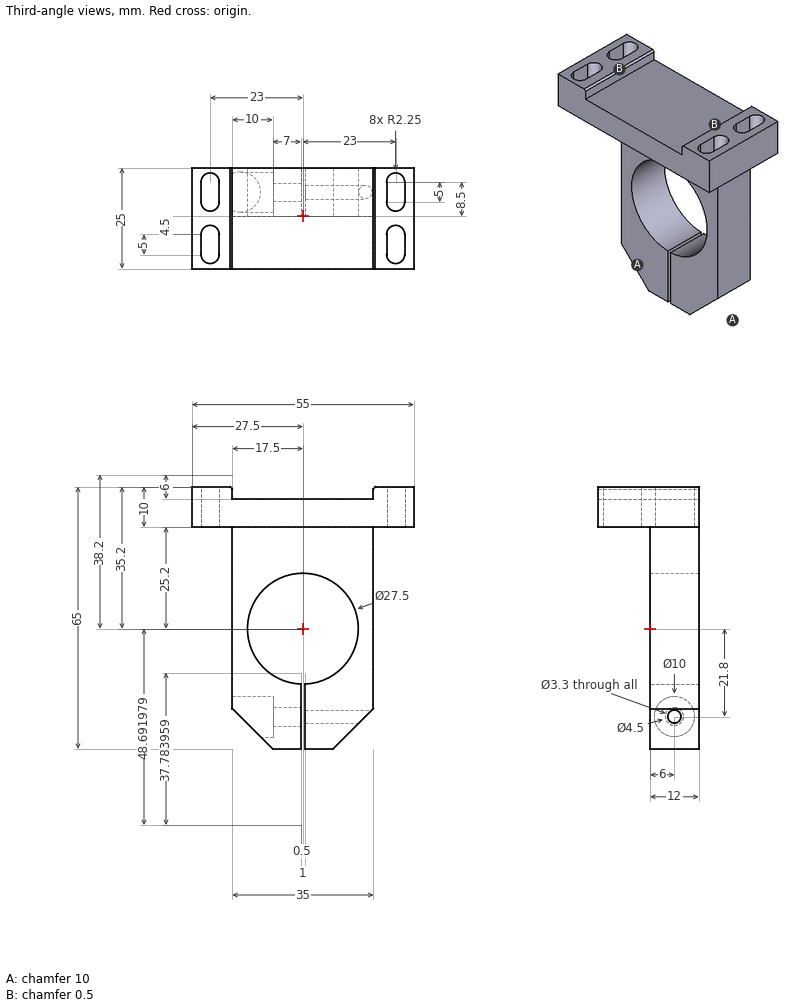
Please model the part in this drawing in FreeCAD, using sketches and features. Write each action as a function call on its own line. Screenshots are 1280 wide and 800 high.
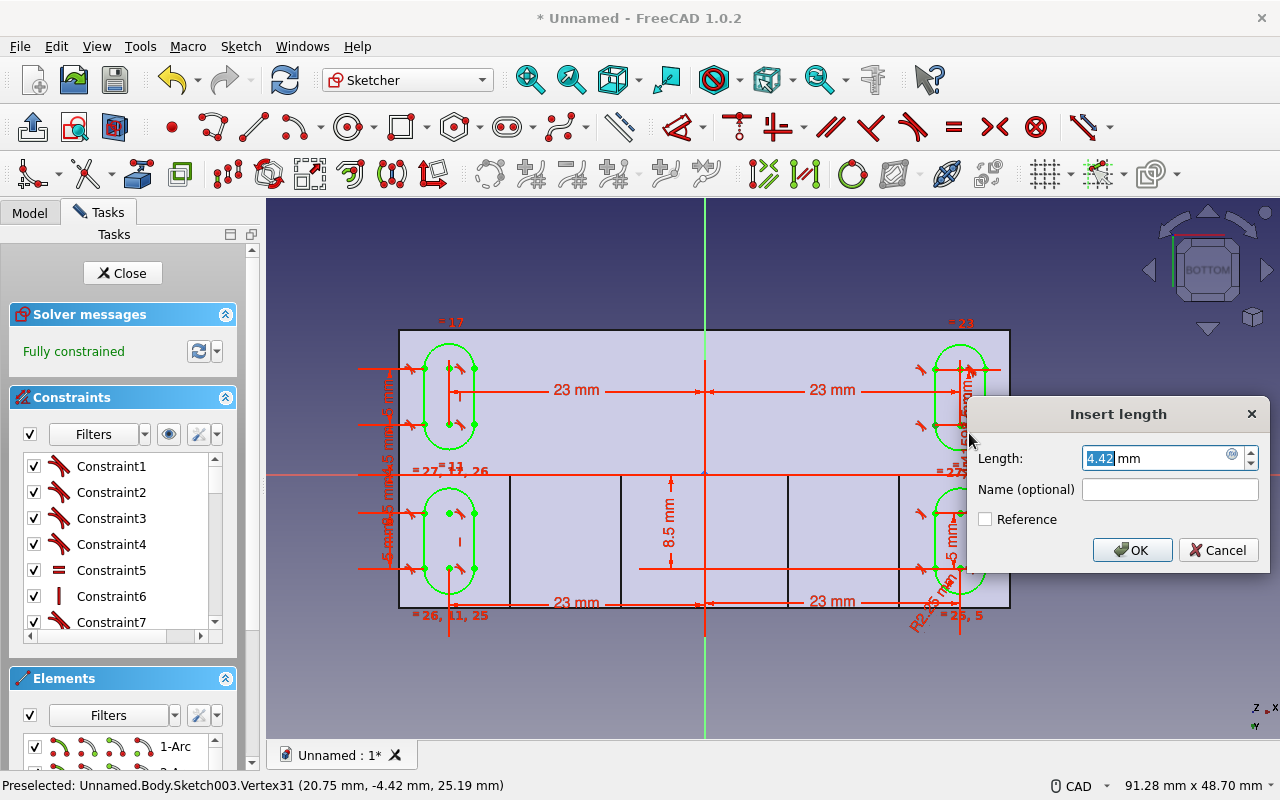
text(4.5)
key(Return)
key(Escape)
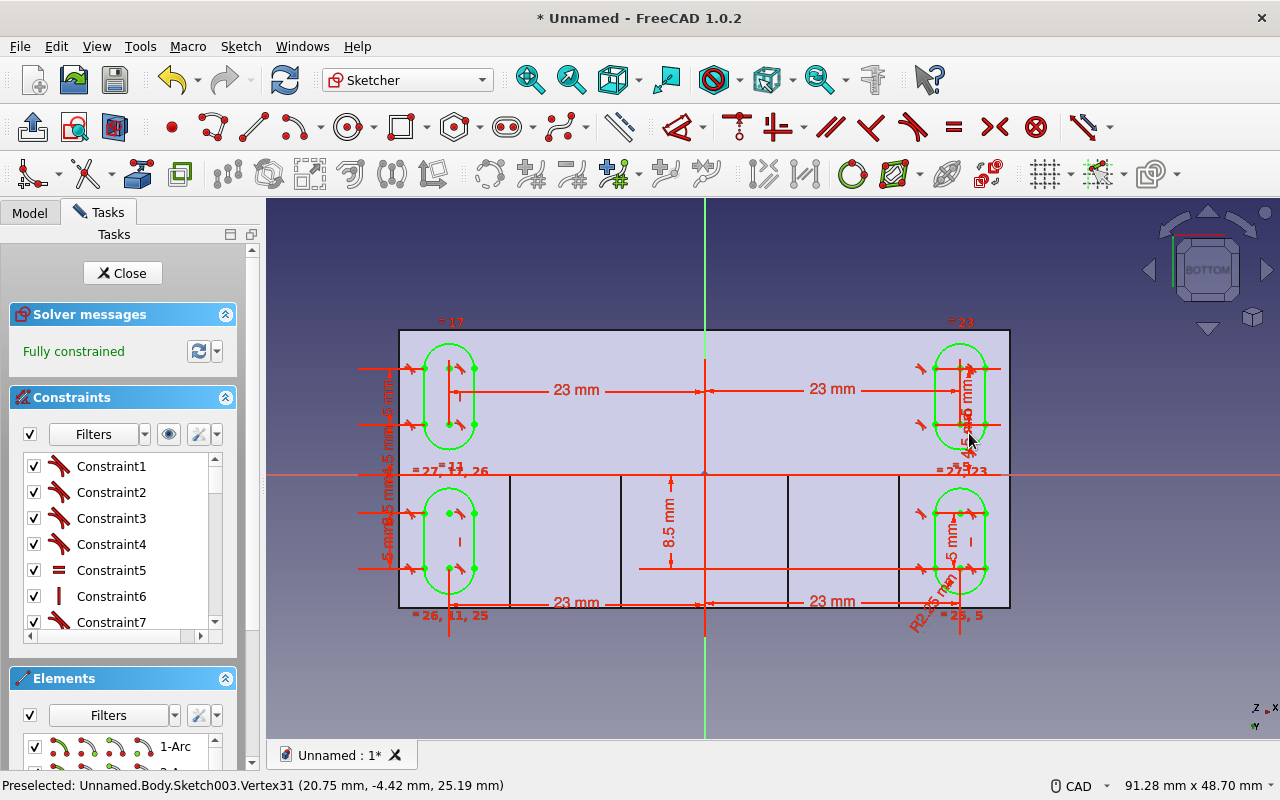
click(123, 273)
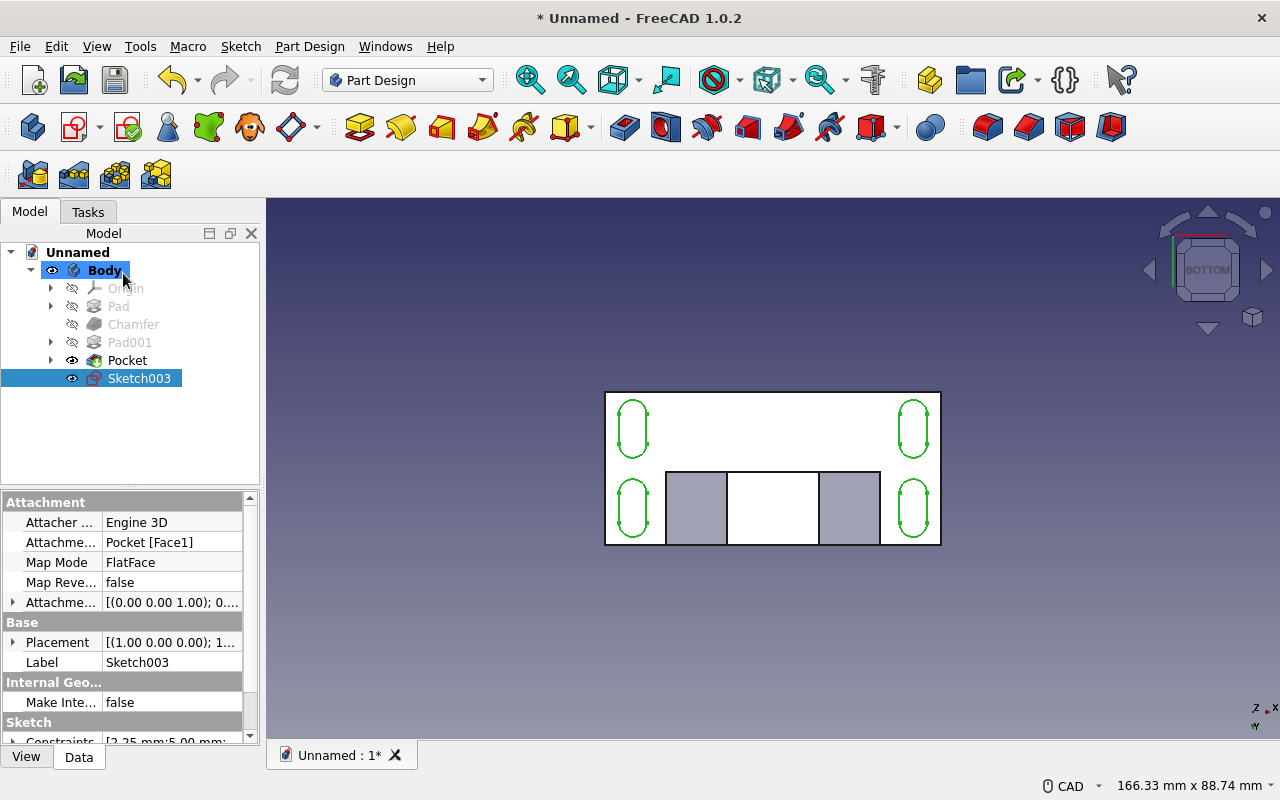
click(625, 128)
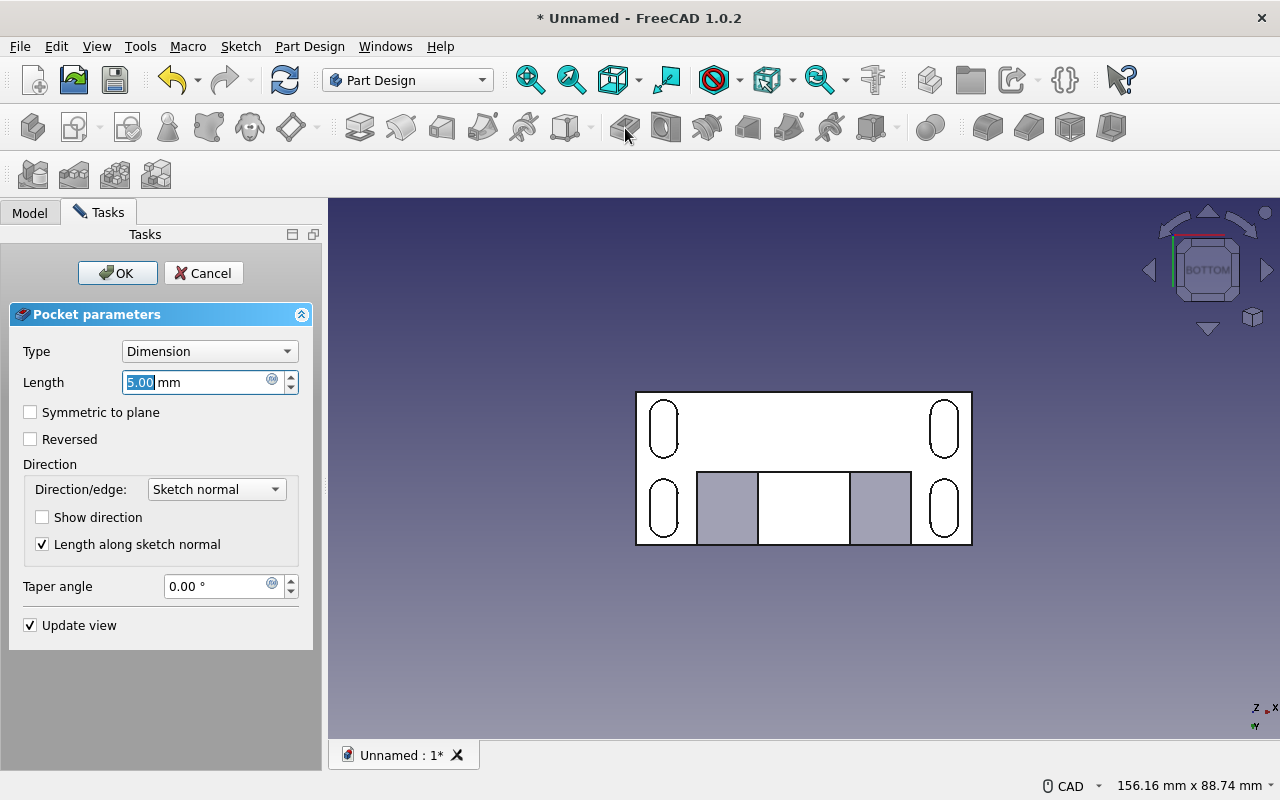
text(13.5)
key(Tab)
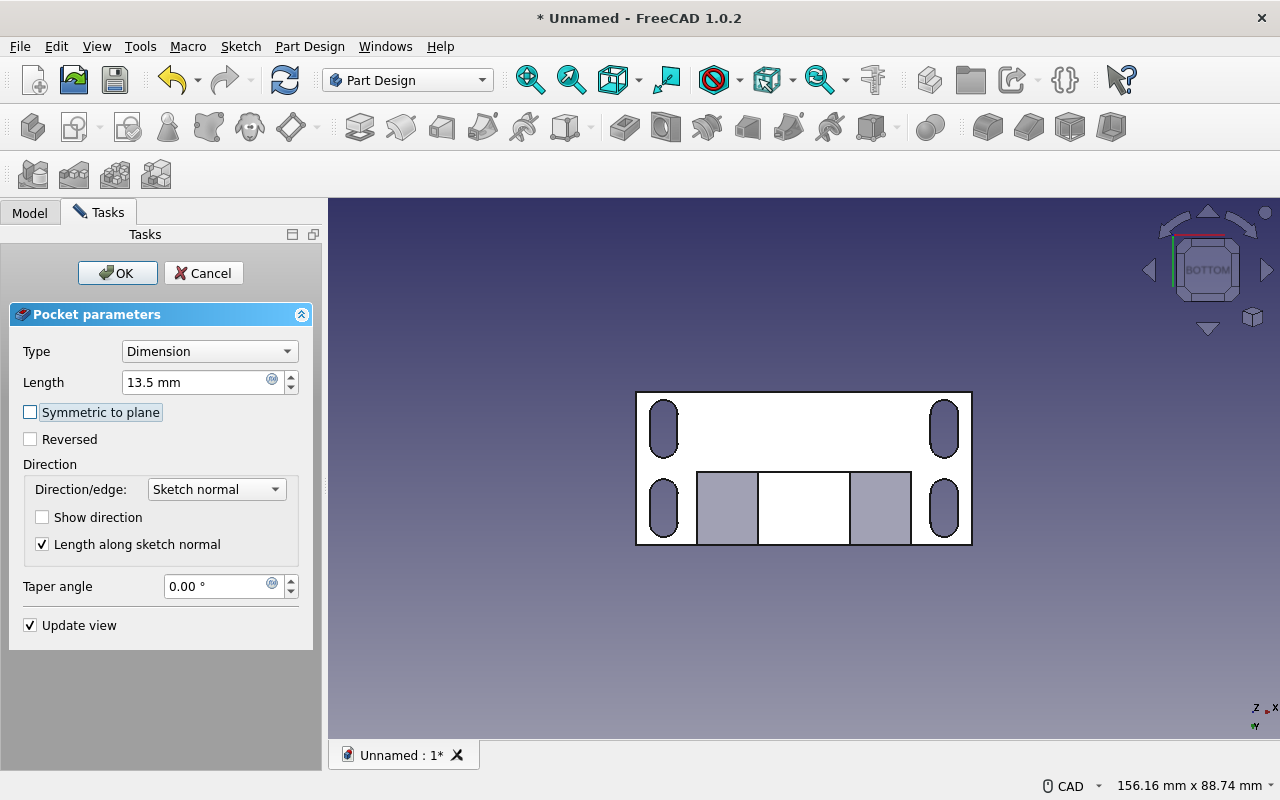
click(118, 273)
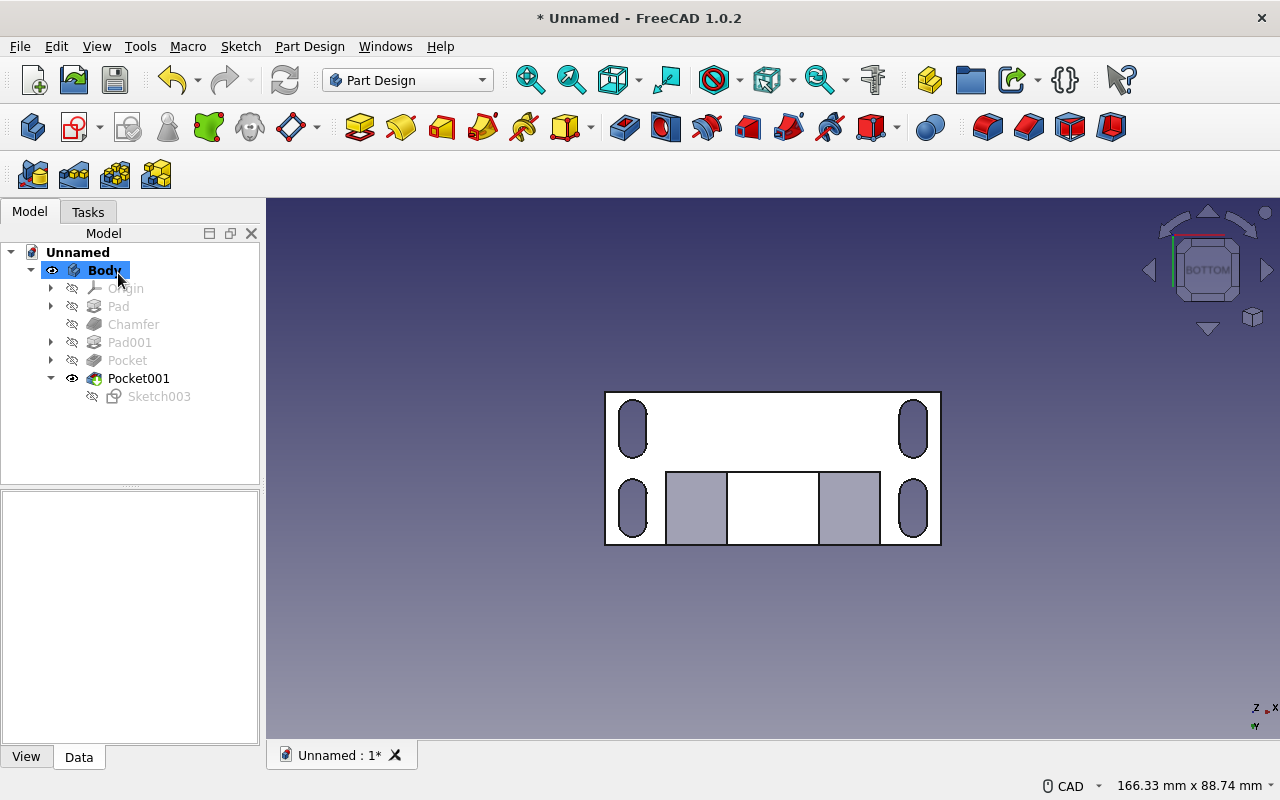
key(v)
key(f)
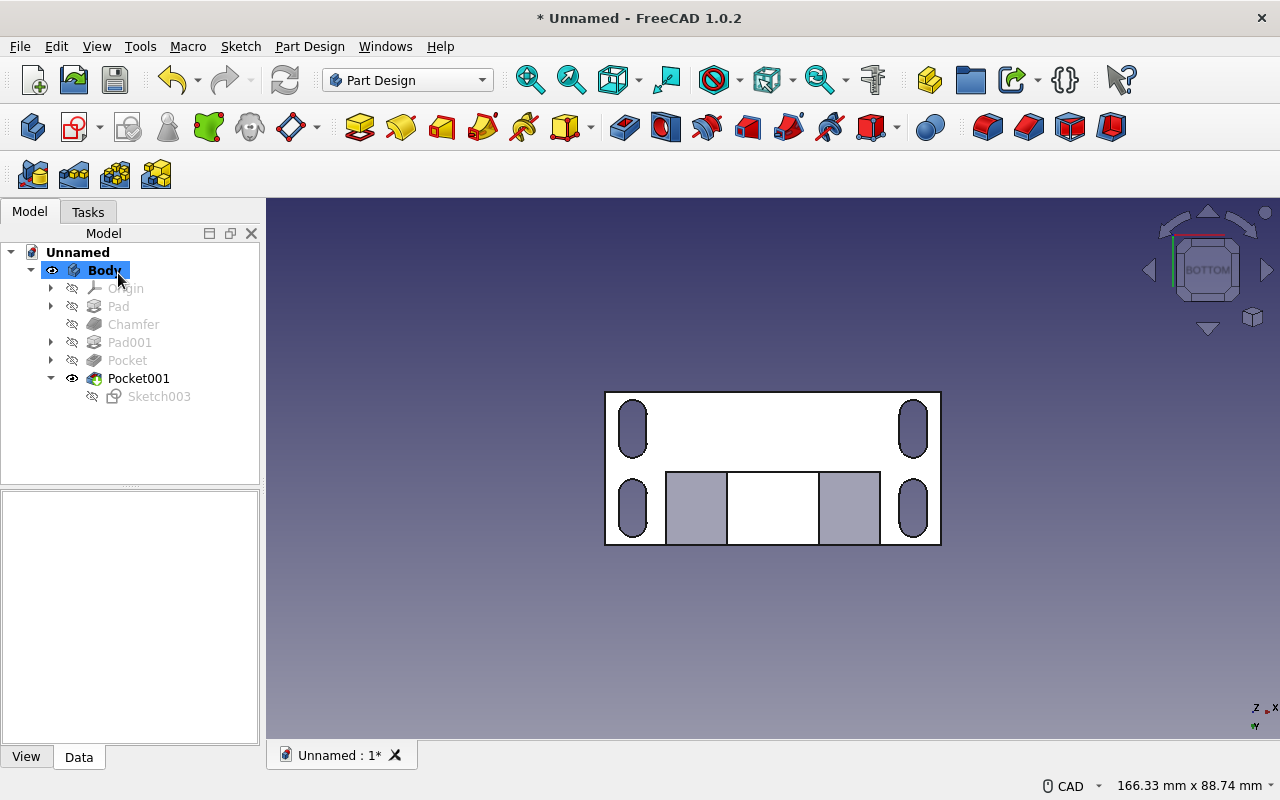
key(0)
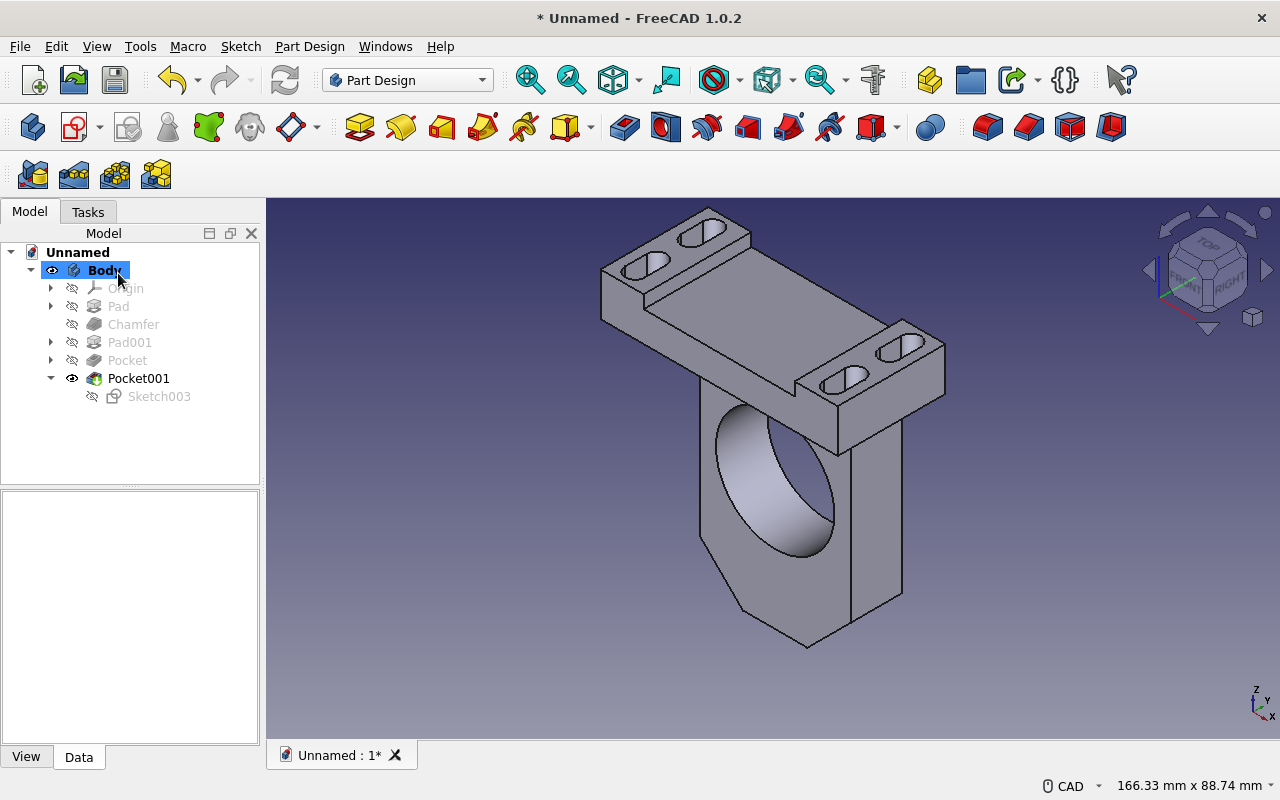
click(698, 262)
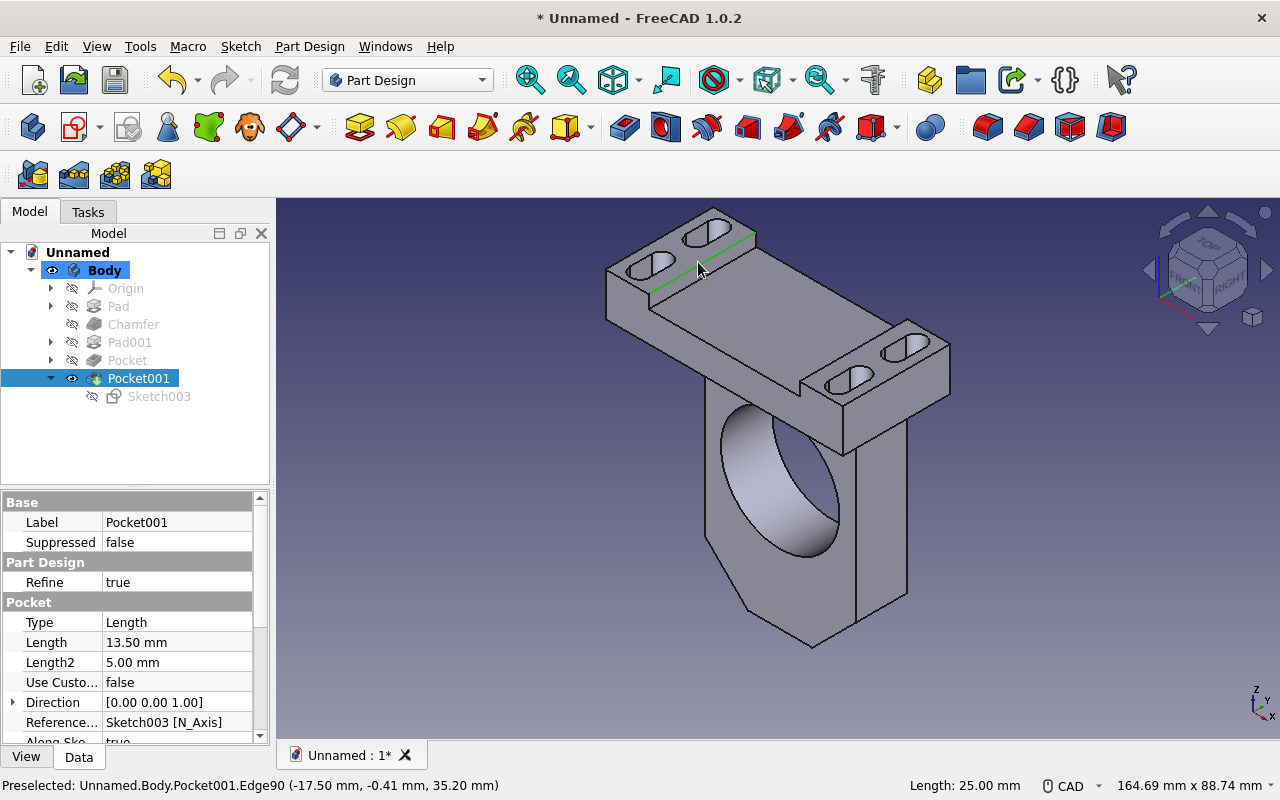
key(2)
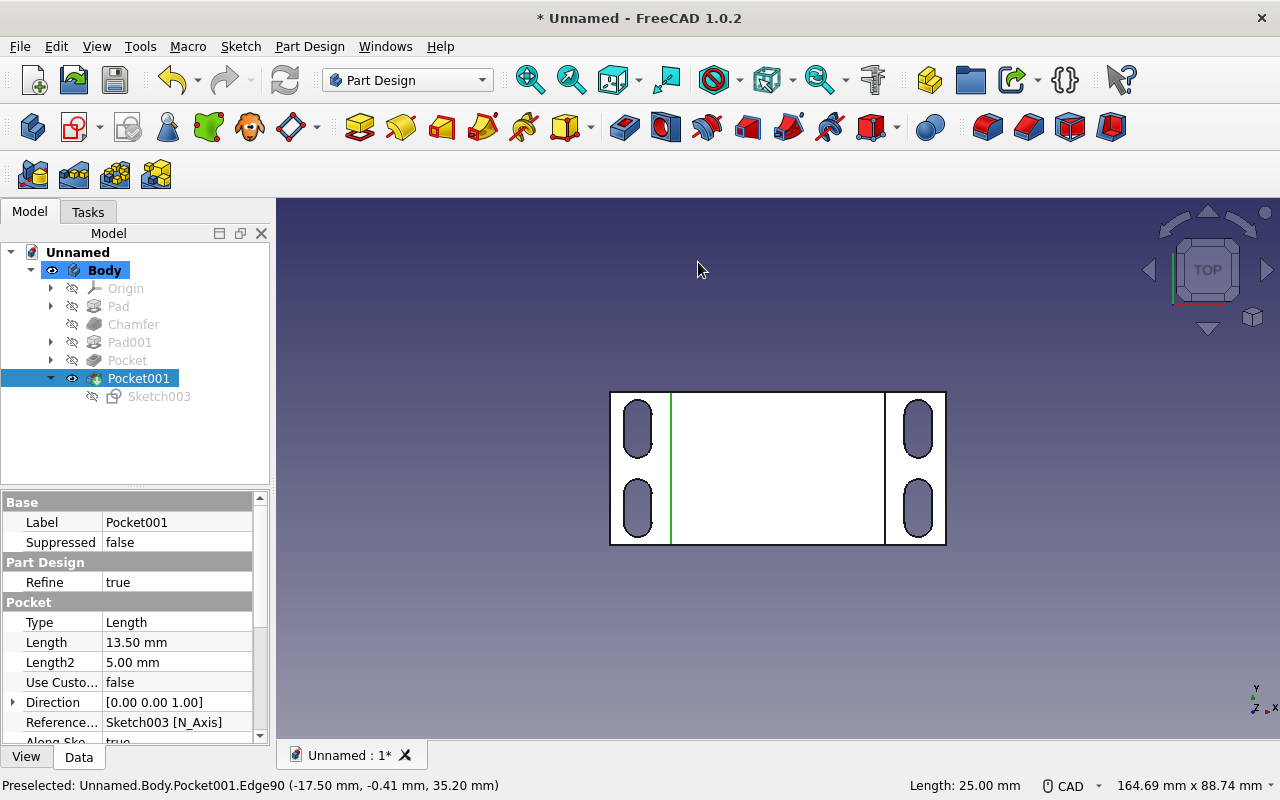
key(v)
key(f)